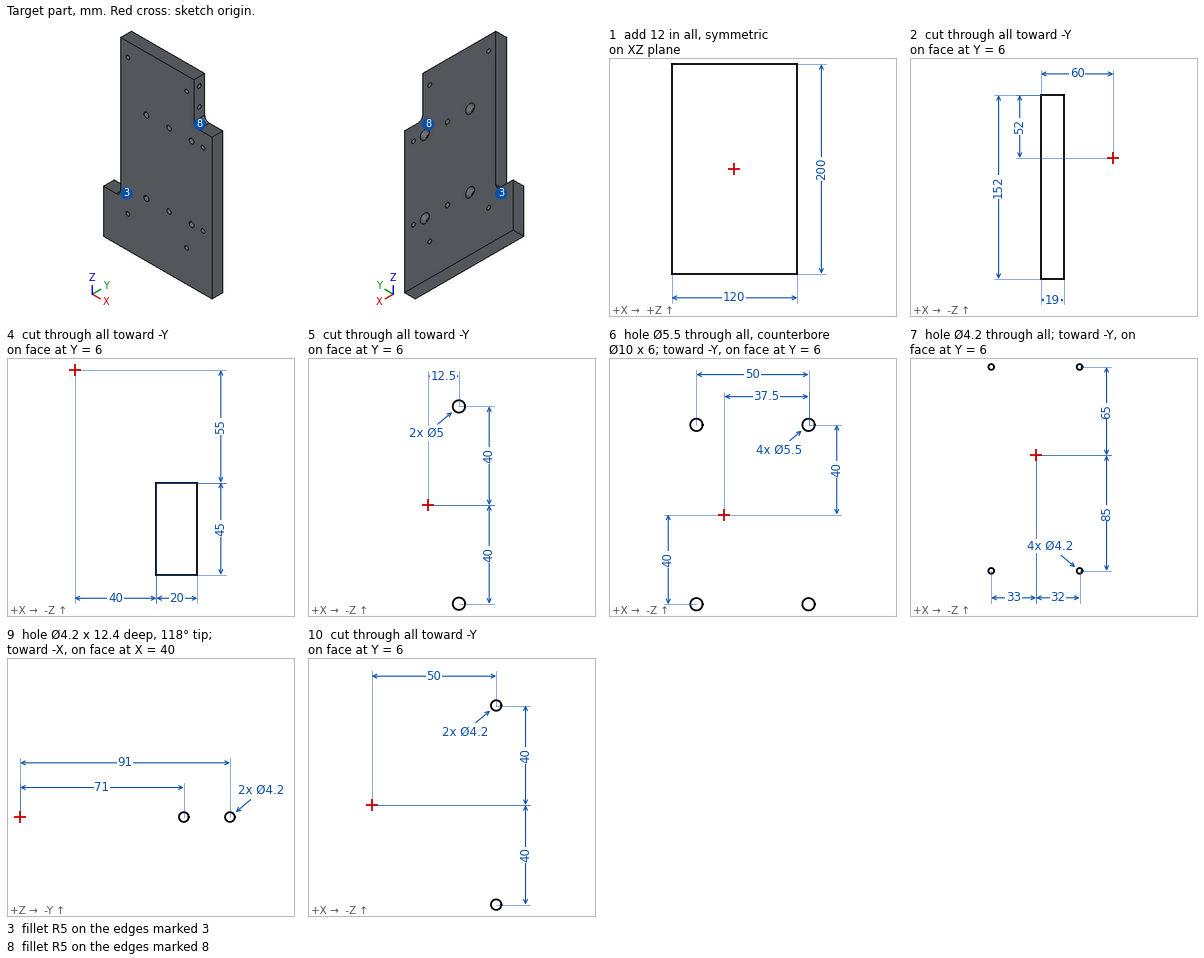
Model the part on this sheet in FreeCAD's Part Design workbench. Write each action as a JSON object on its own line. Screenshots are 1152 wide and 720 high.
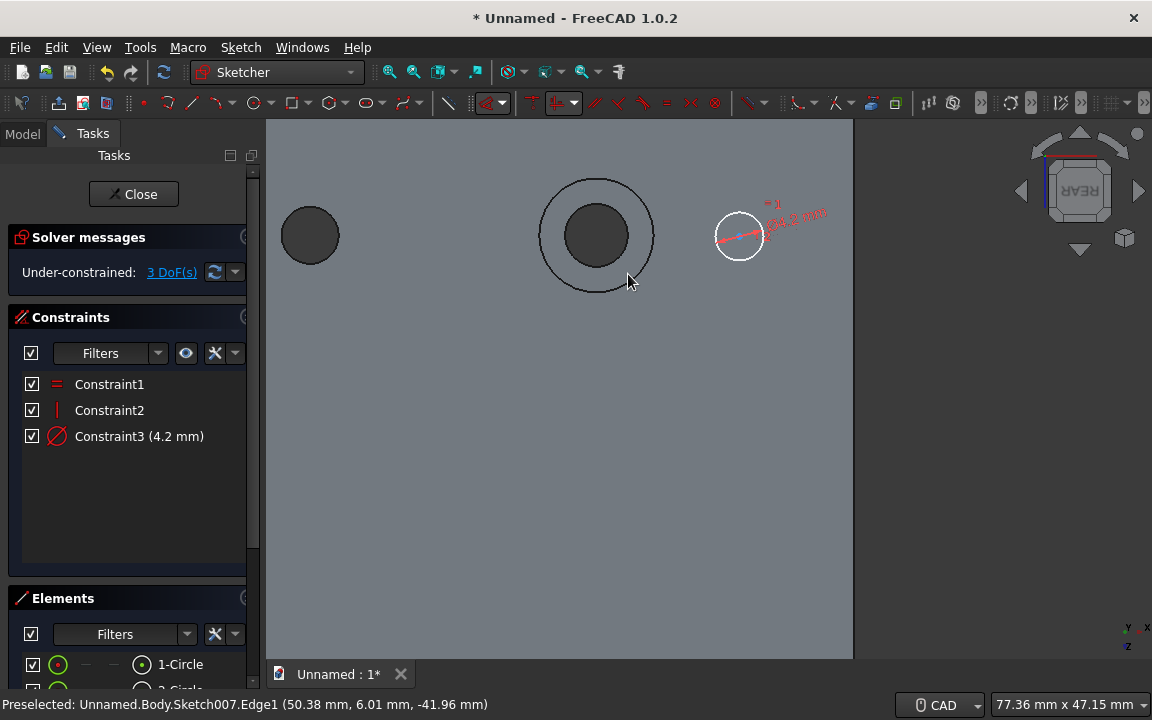
{"action": "left_click", "coordinate": [739, 236]}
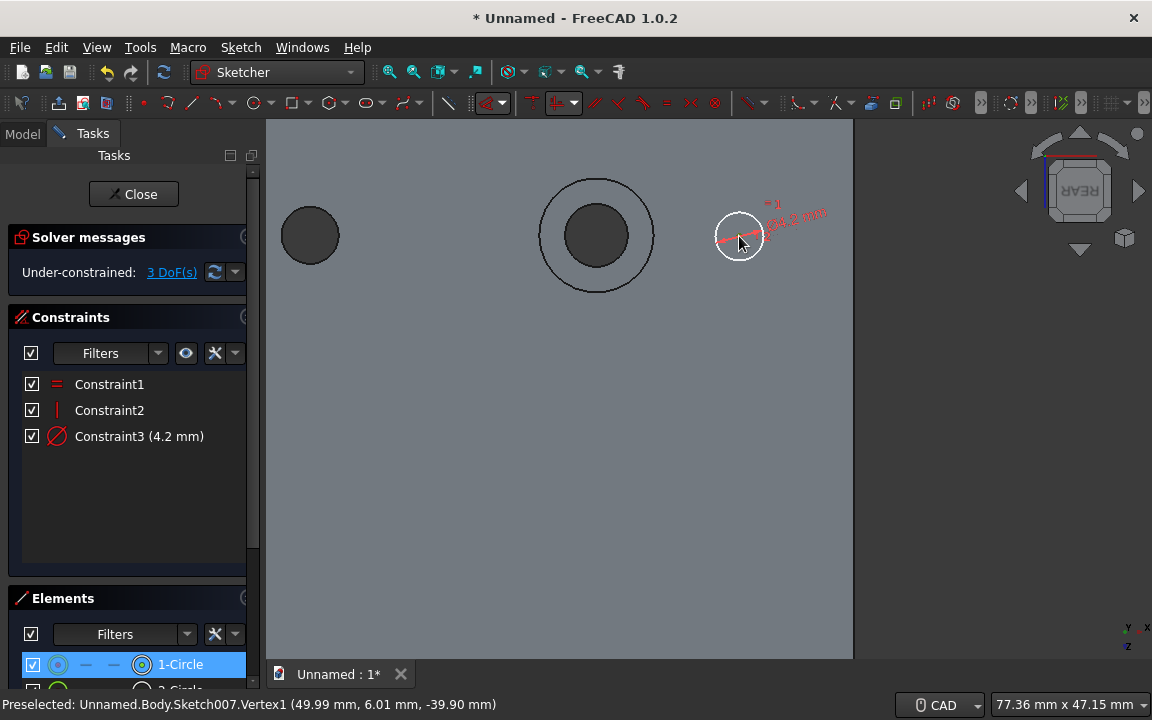
{"action": "left_click", "coordinate": [504, 104]}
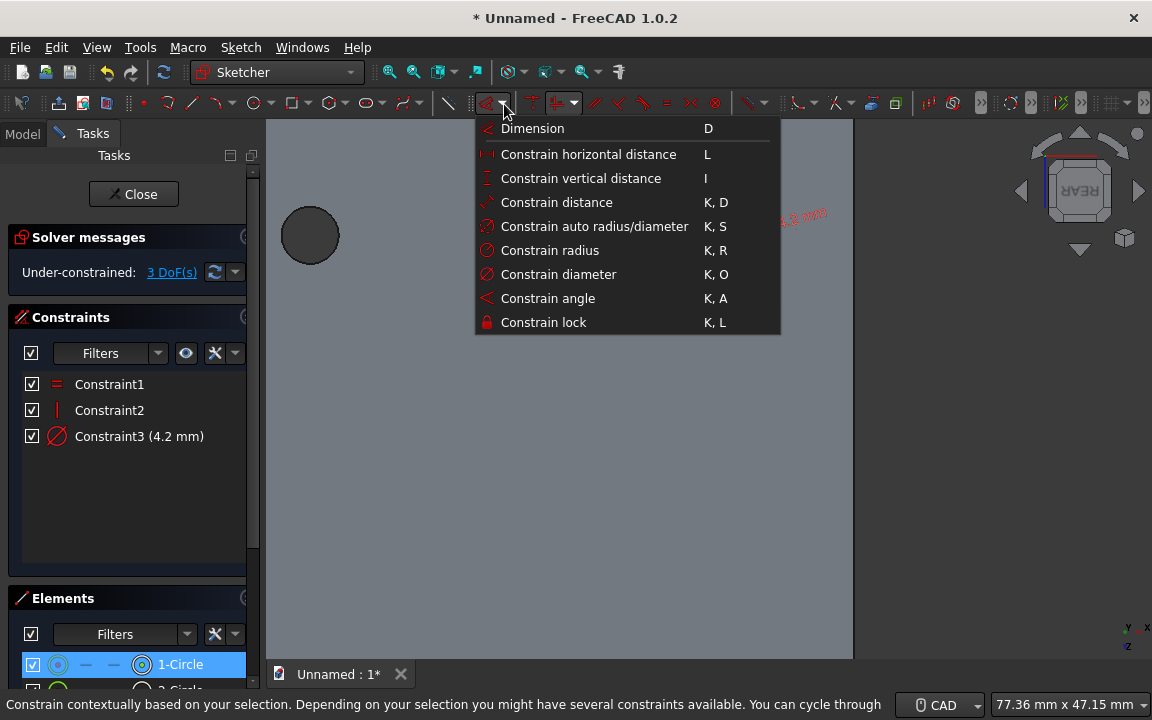
{"action": "left_click", "coordinate": [628, 154]}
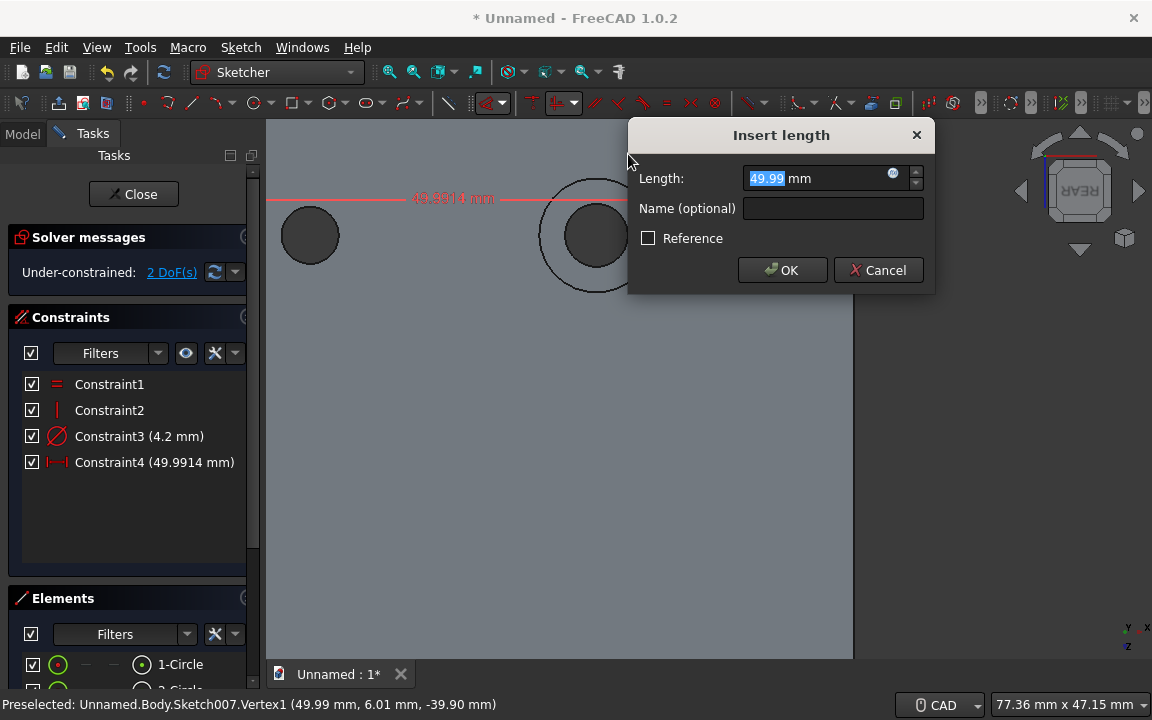
{"action": "type", "text": "50"}
{"action": "key", "text": "Return"}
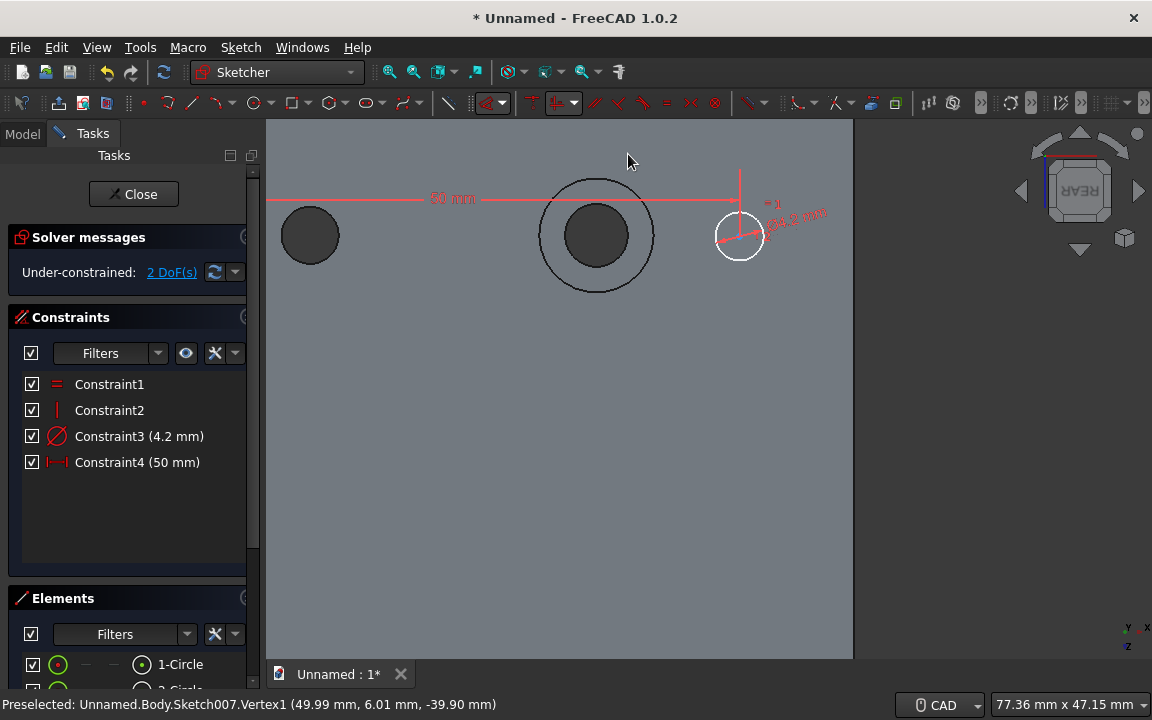
{"action": "left_click", "coordinate": [740, 236]}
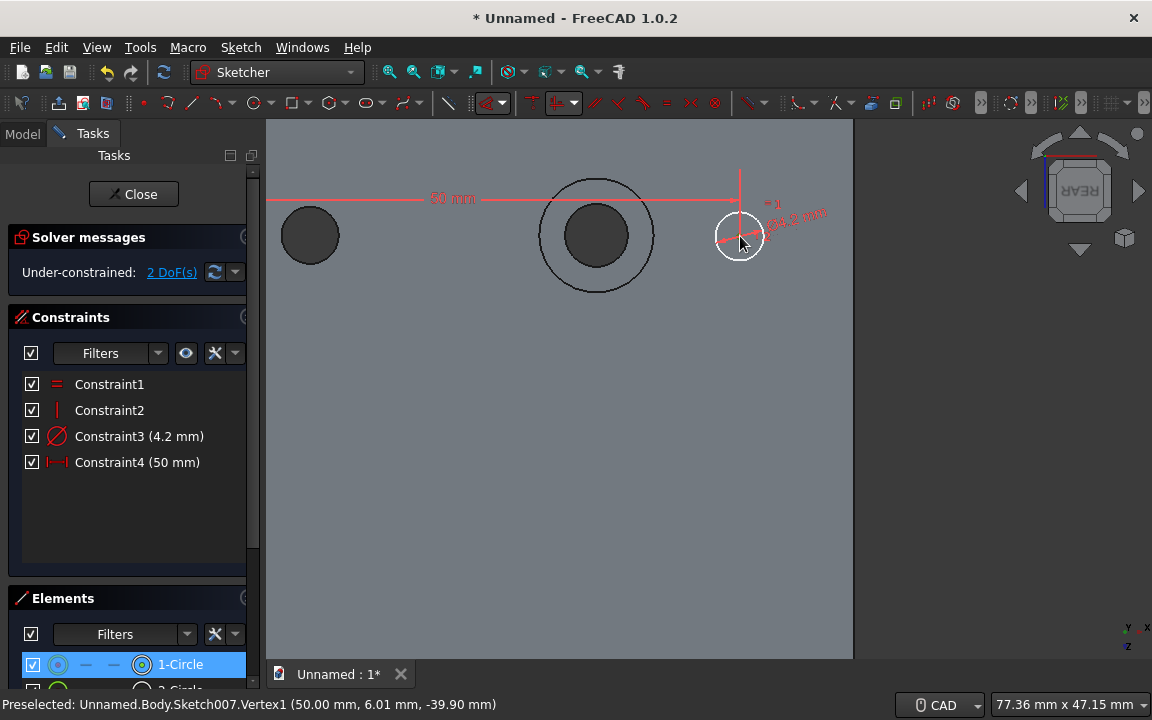
{"action": "left_click", "coordinate": [504, 104]}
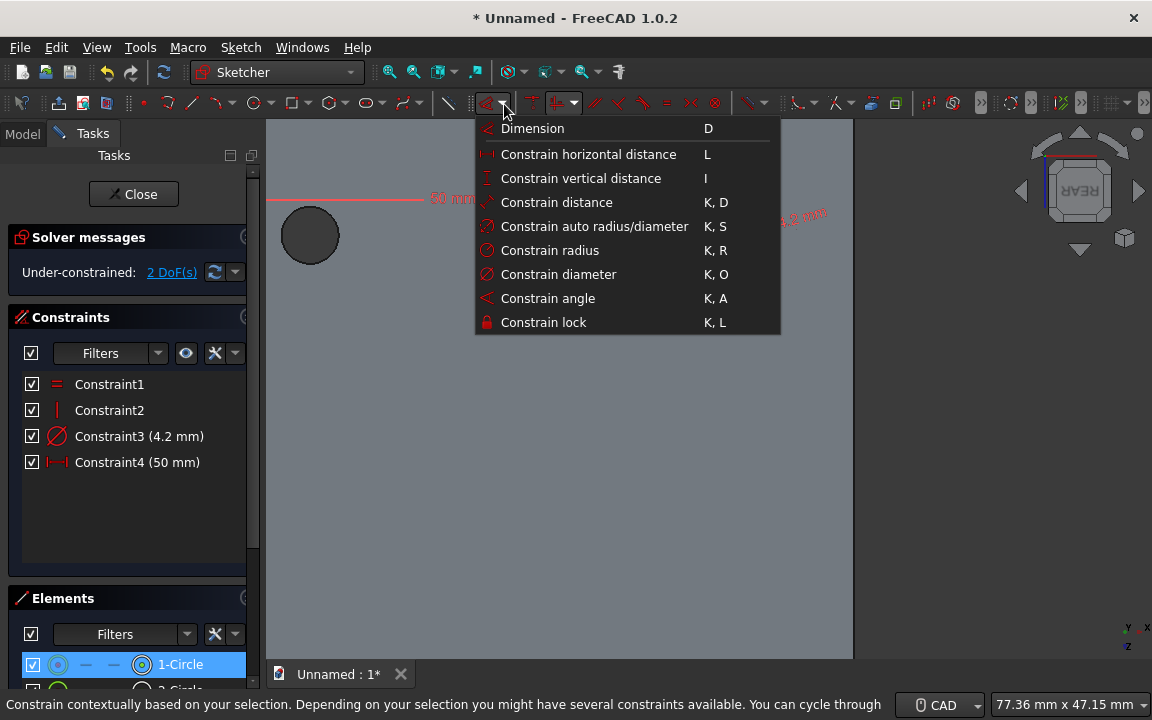
{"action": "left_click", "coordinate": [628, 178]}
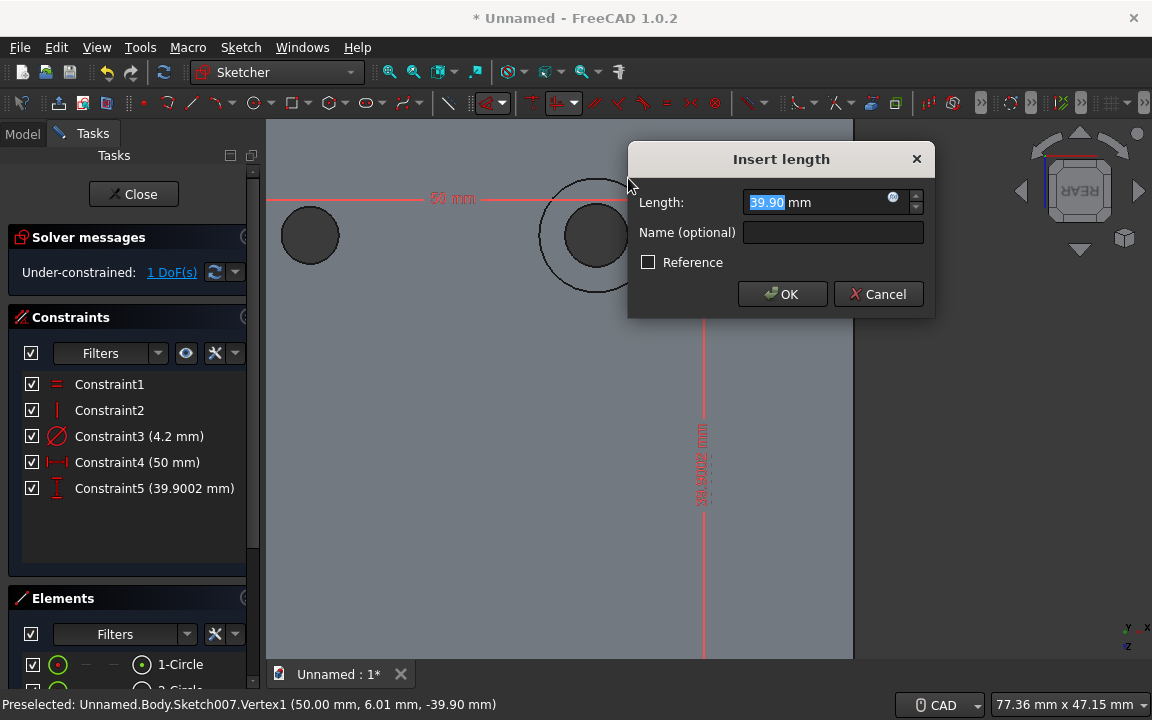
{"action": "type", "text": "40"}
{"action": "key", "text": "Return"}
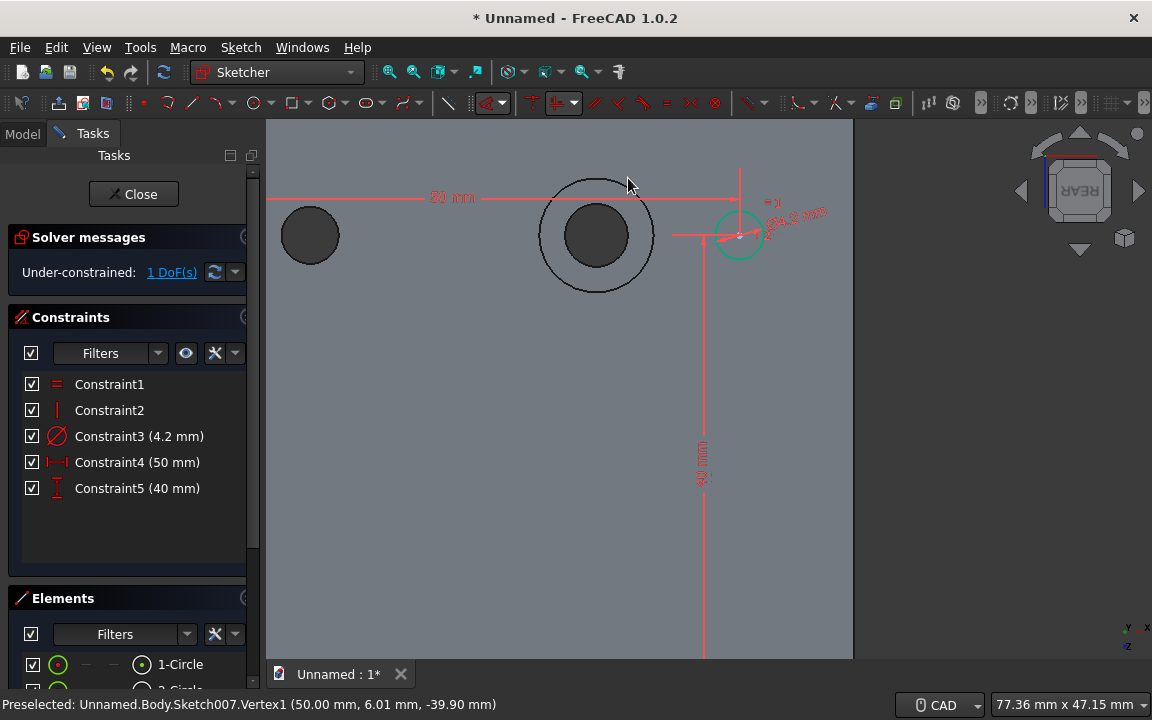
{"action": "scroll", "coordinate": [742, 212], "scroll_direction": "down", "scroll_amount": 5}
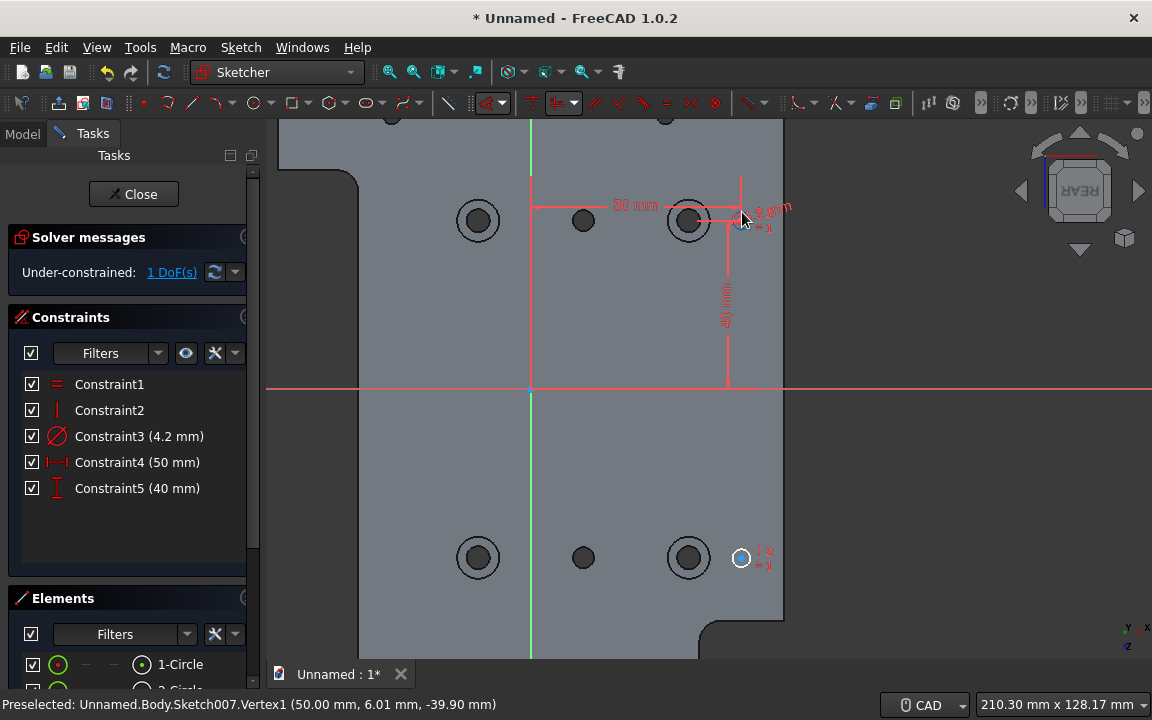
{"action": "left_click", "coordinate": [741, 558]}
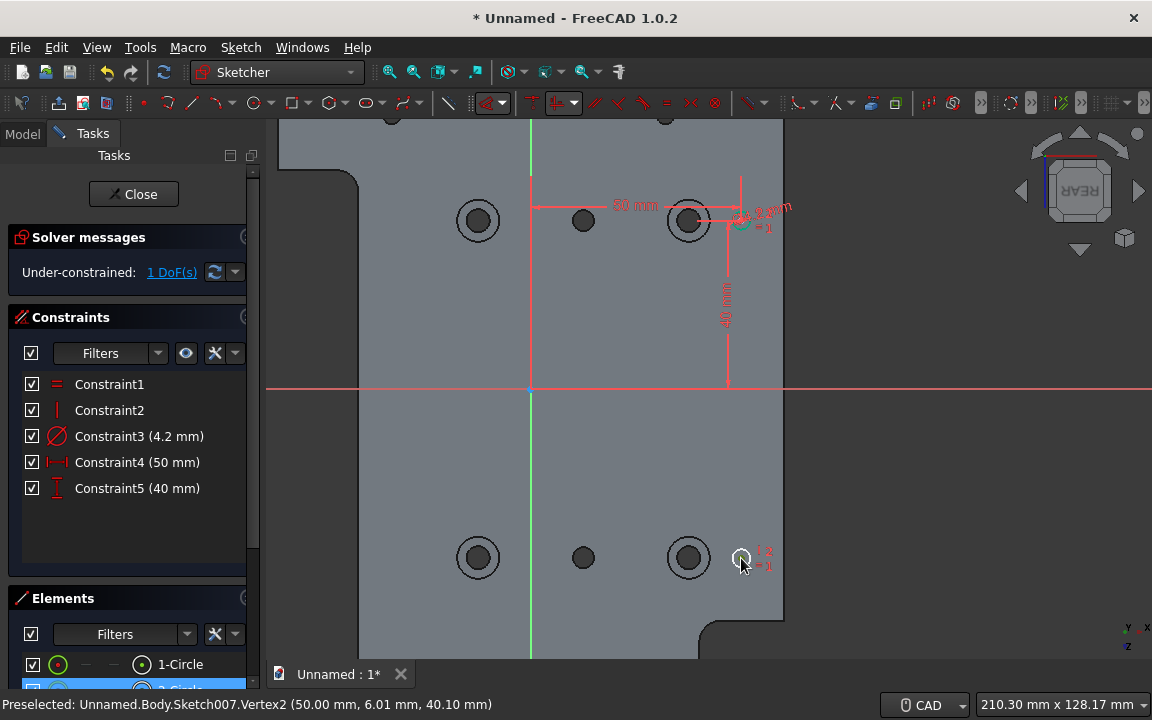
{"action": "left_click", "coordinate": [504, 104]}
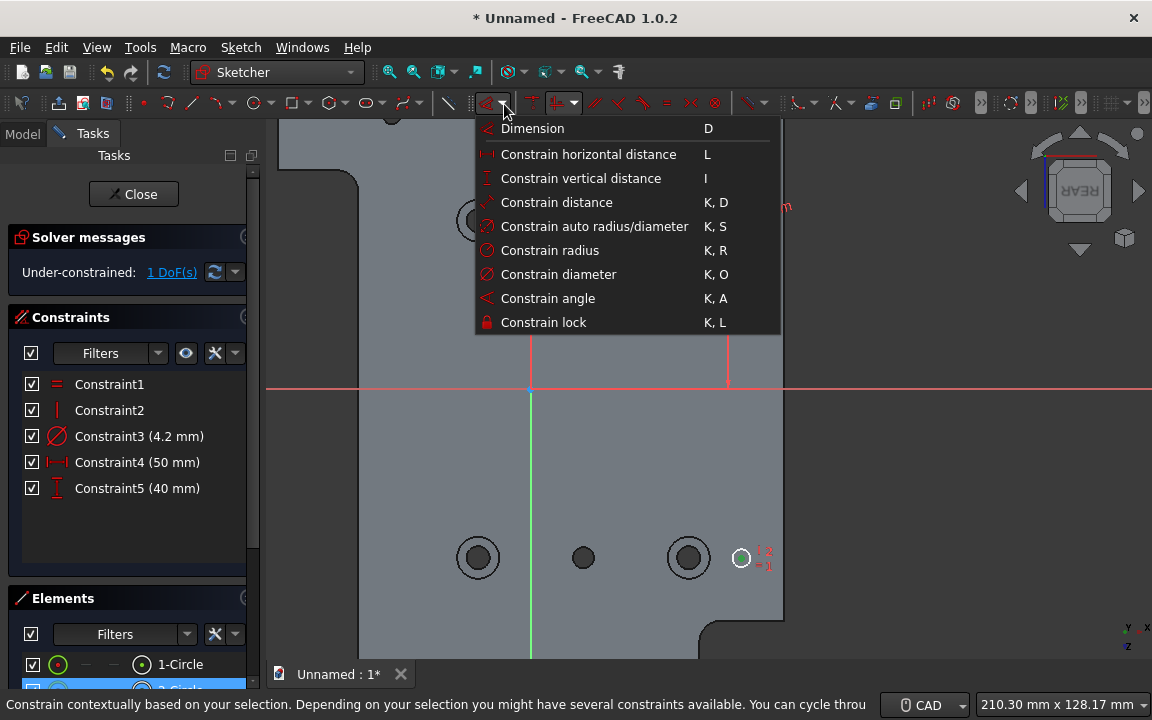
{"action": "left_click", "coordinate": [628, 178]}